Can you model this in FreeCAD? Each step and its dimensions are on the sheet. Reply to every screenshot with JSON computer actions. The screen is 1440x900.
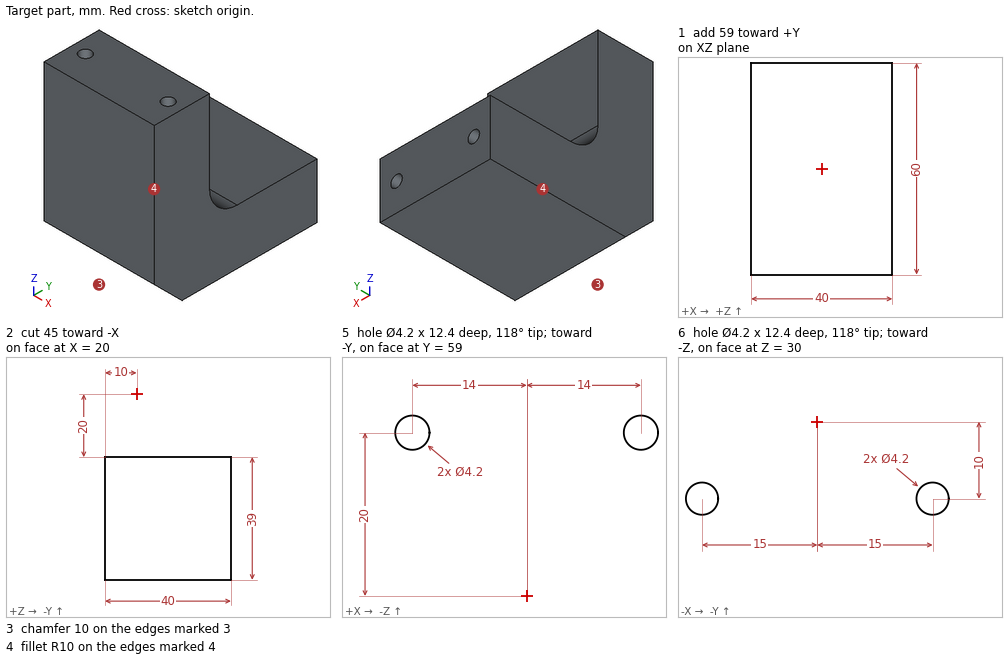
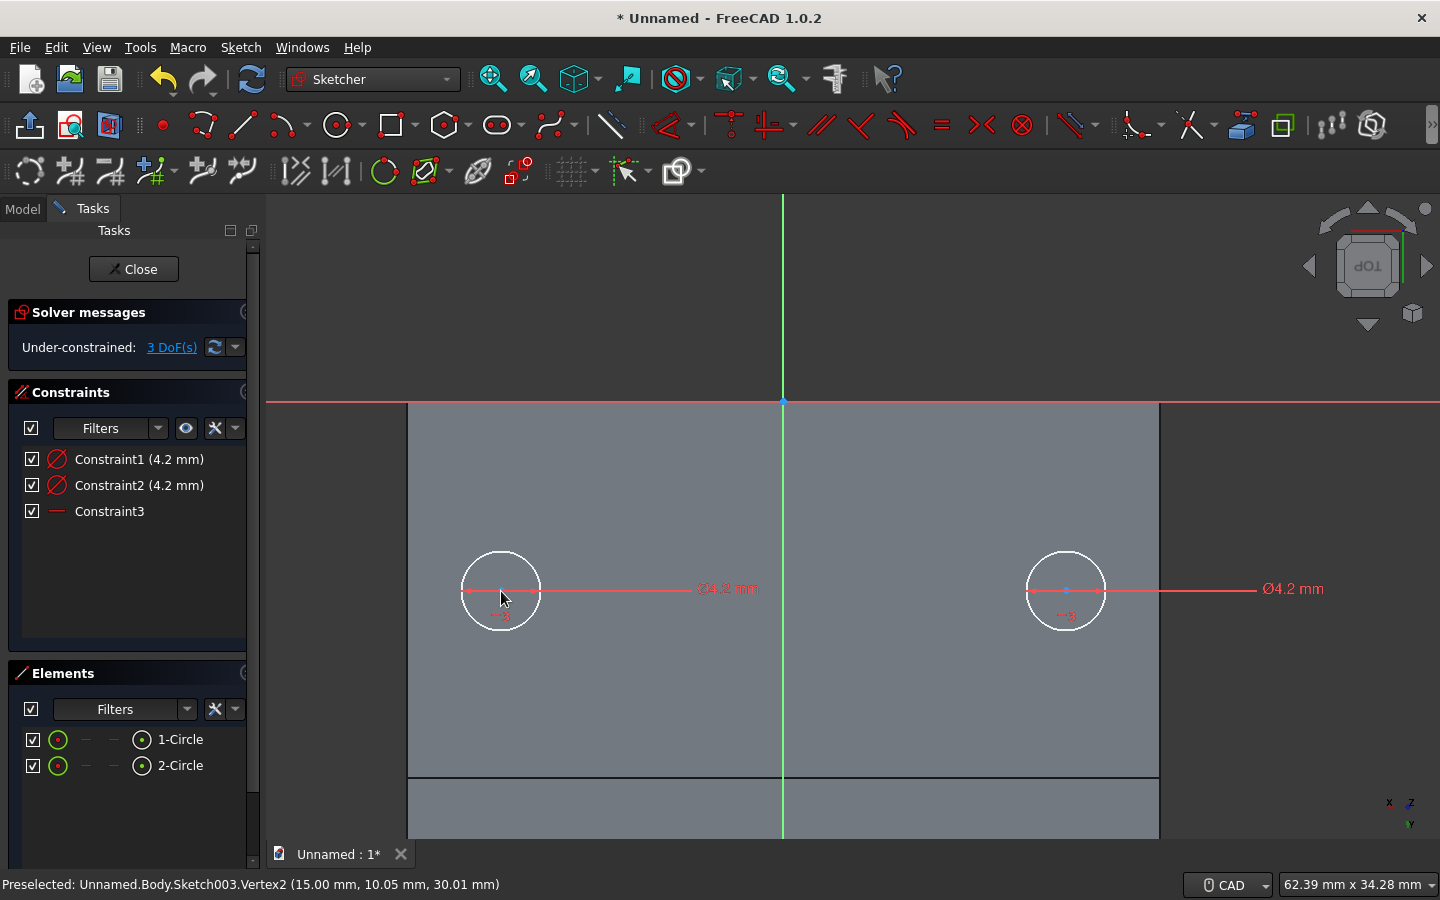
{"action": "left_click", "coordinate": [666, 126]}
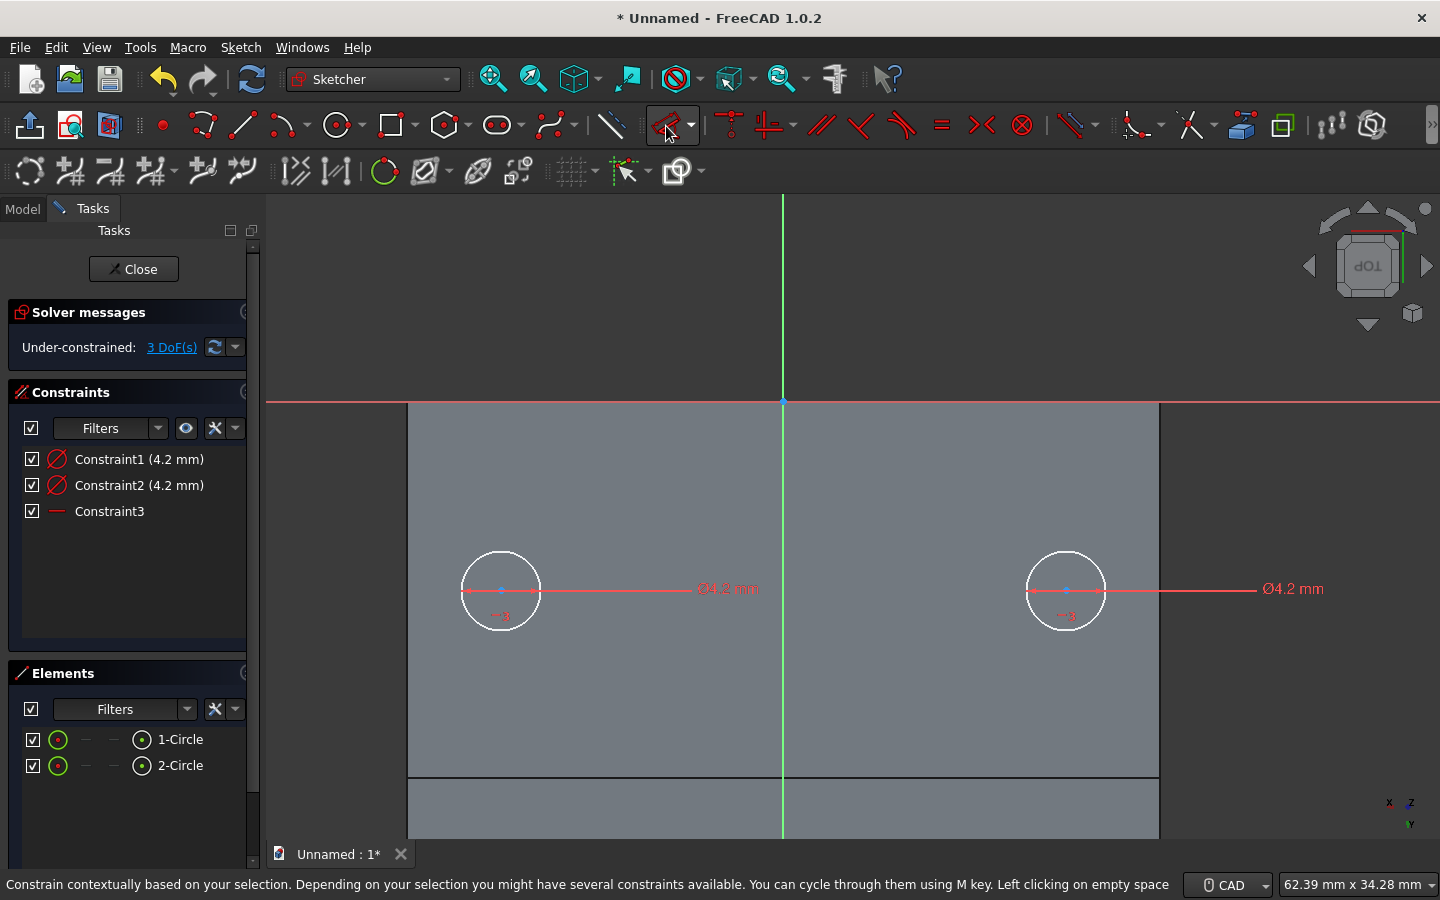
{"action": "left_click", "coordinate": [1066, 591]}
{"action": "left_click", "coordinate": [925, 368]}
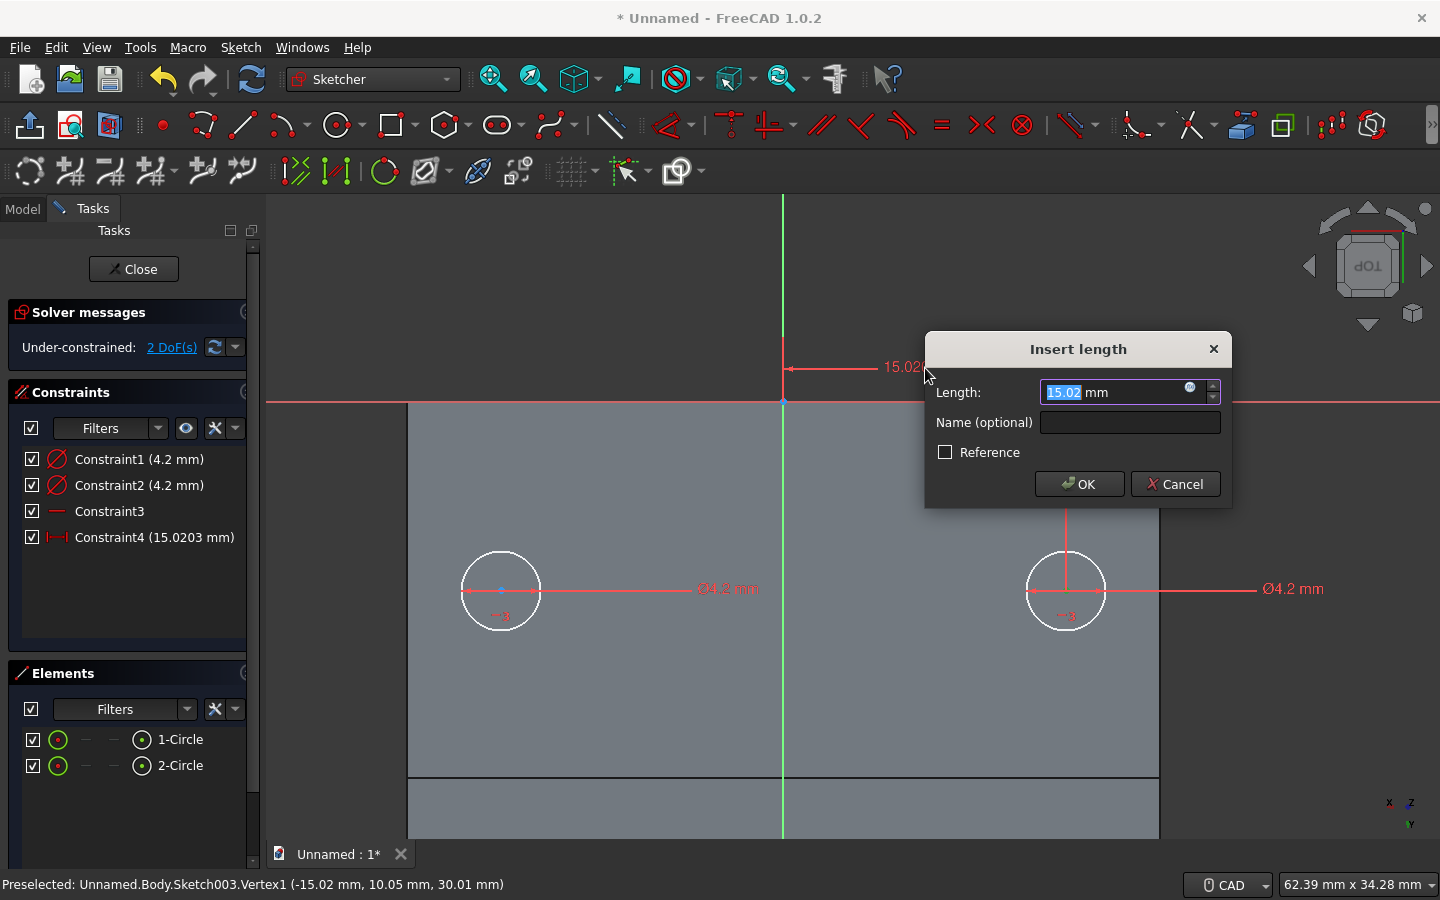
{"action": "type", "text": "15"}
{"action": "key", "text": "Return"}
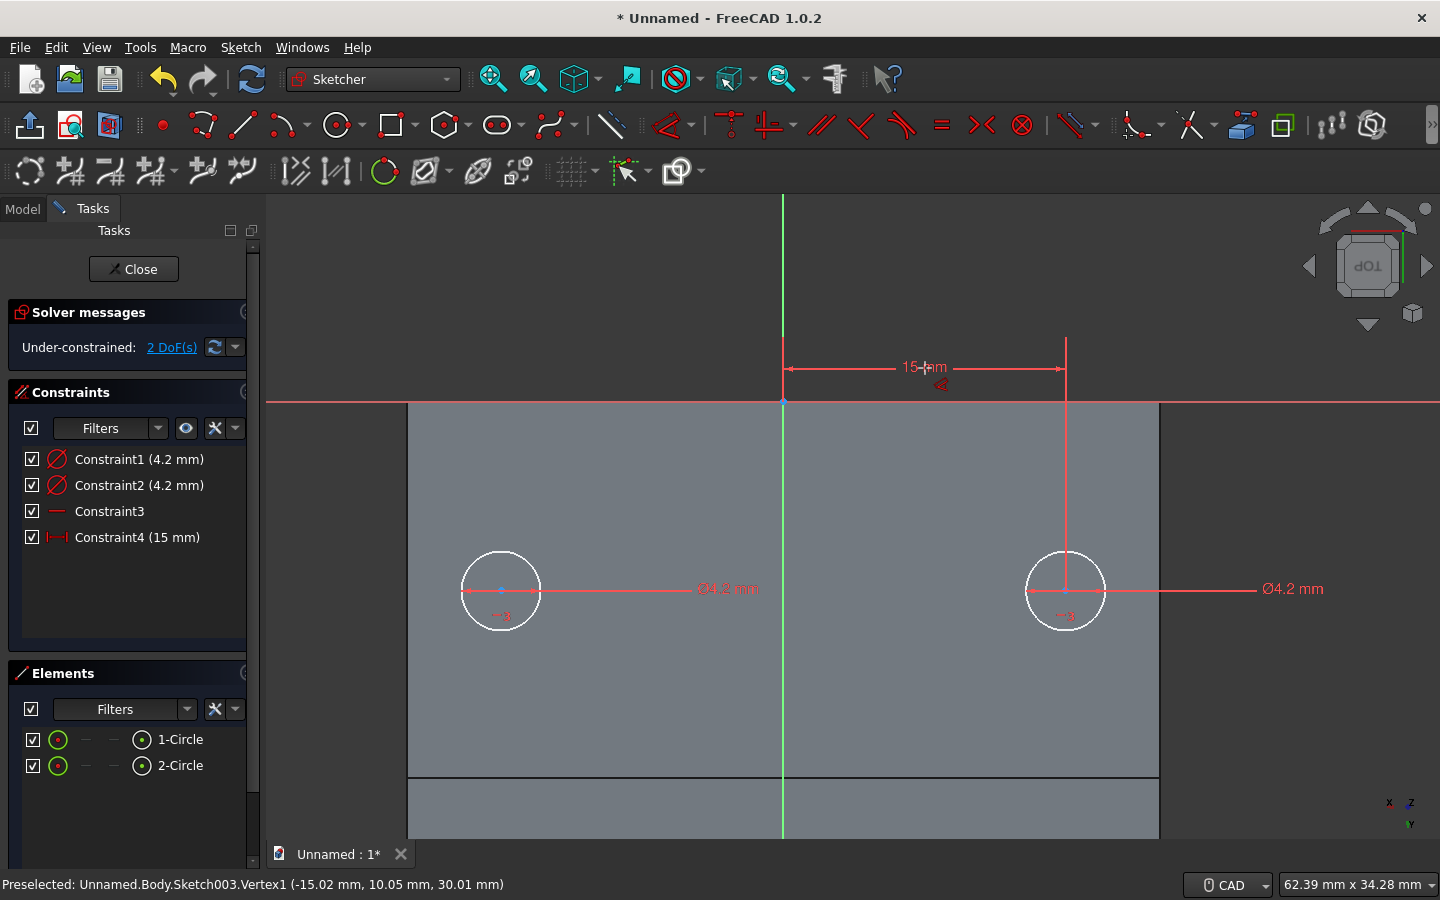
{"action": "left_click", "coordinate": [1066, 591]}
{"action": "left_click", "coordinate": [1100, 496]}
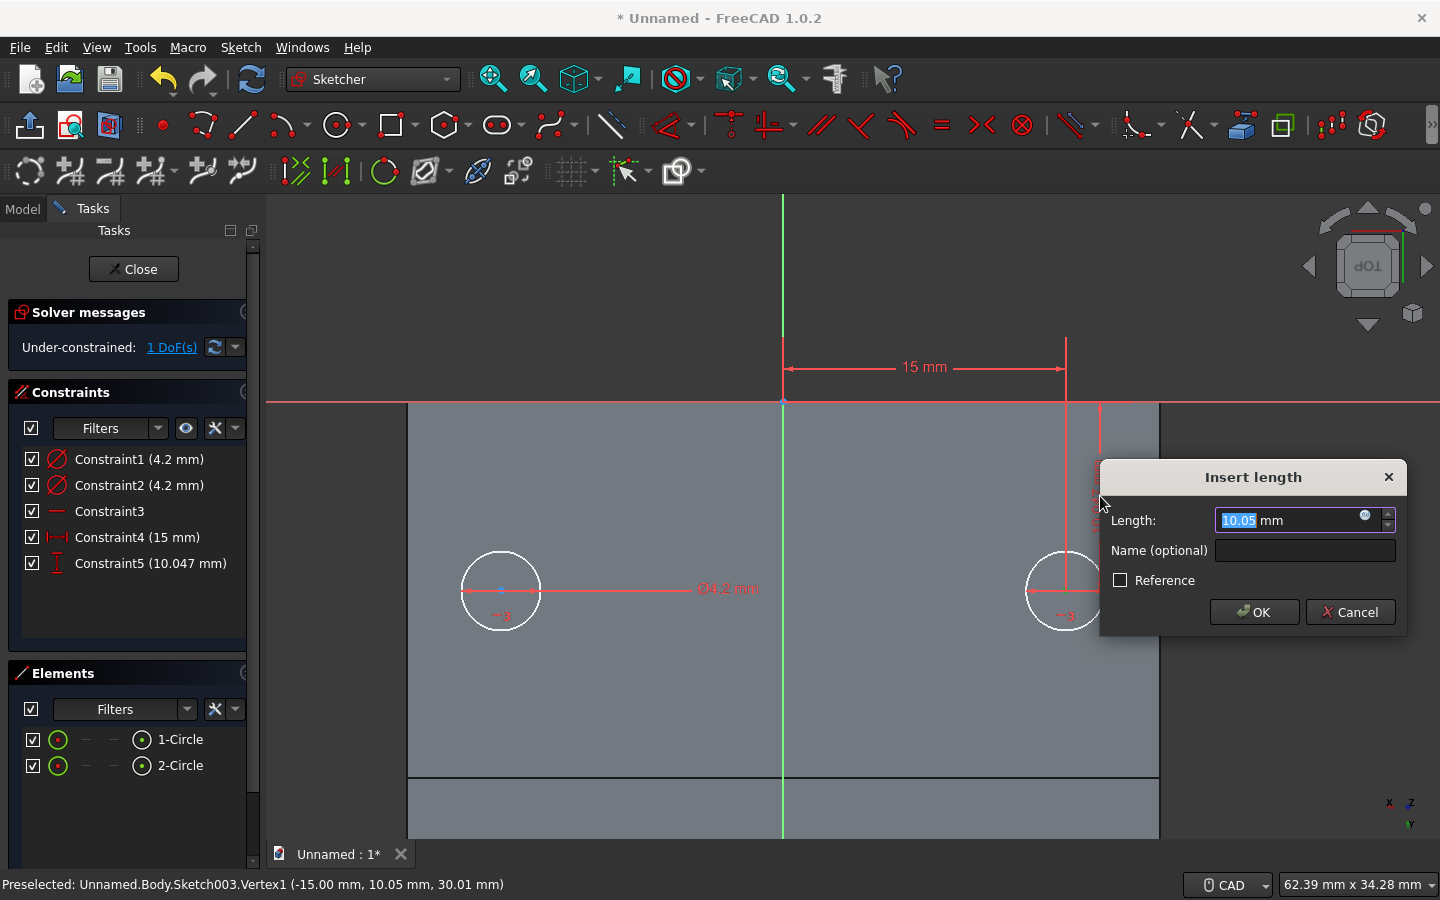
{"action": "type", "text": "10"}
{"action": "key", "text": "Return"}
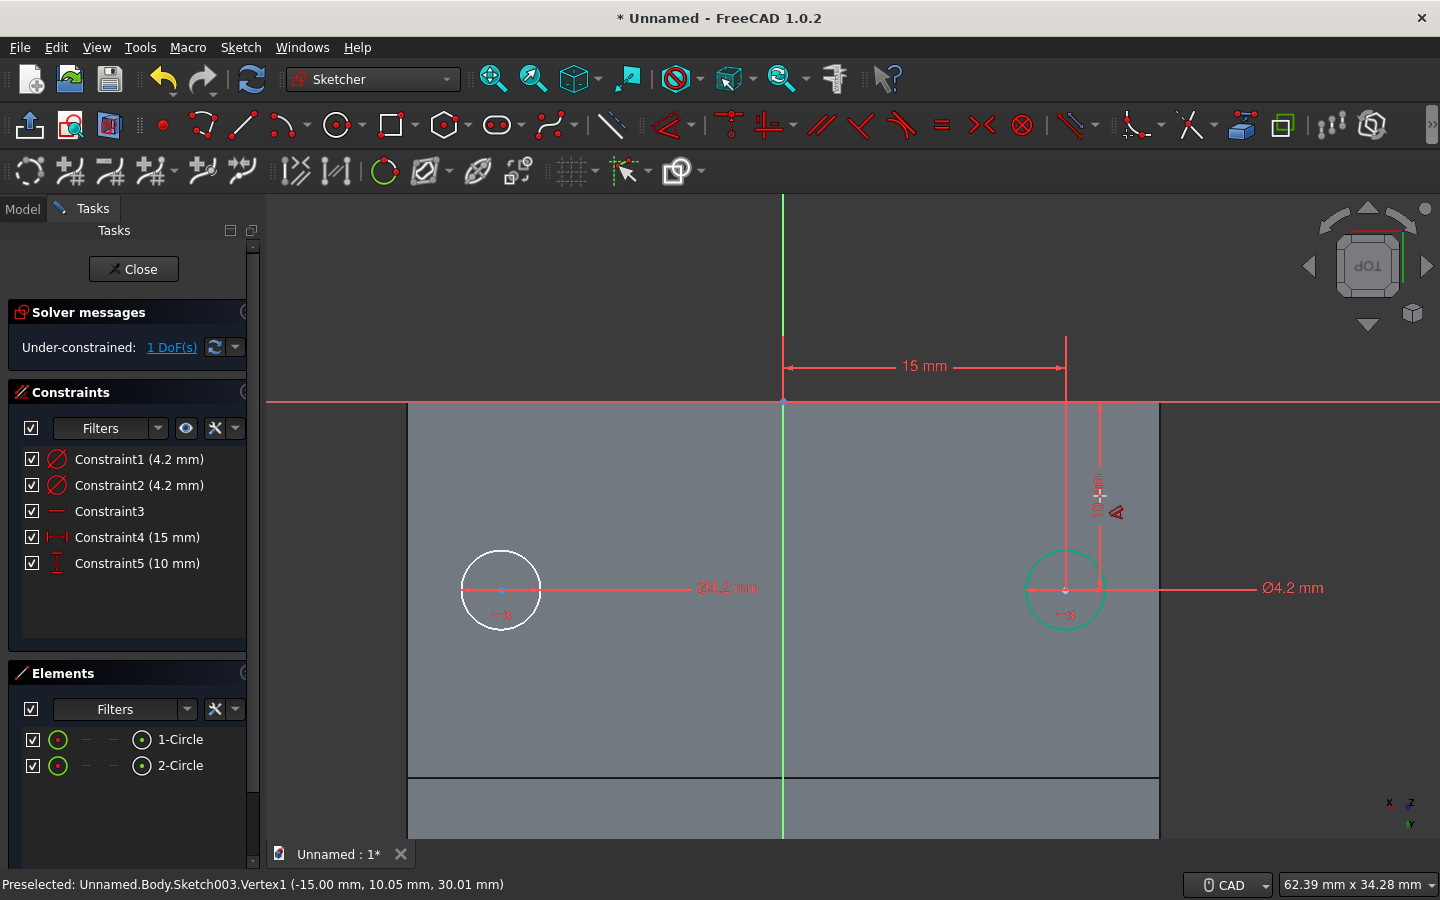
{"action": "left_click", "coordinate": [501, 590]}
{"action": "left_click", "coordinate": [642, 368]}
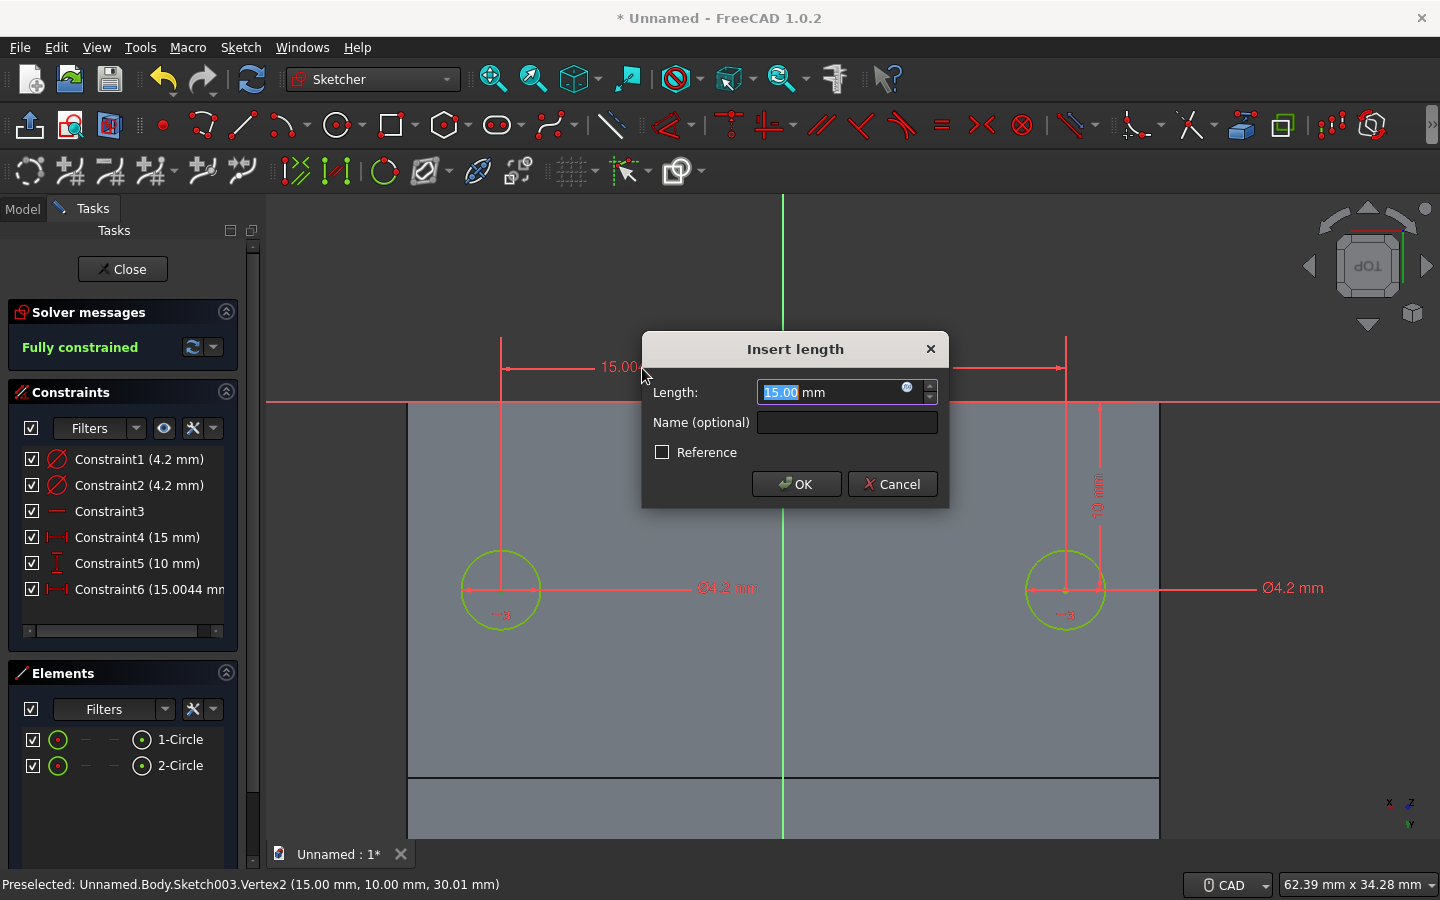
{"action": "type", "text": "15"}
{"action": "key", "text": "Return"}
{"action": "key", "text": "Escape"}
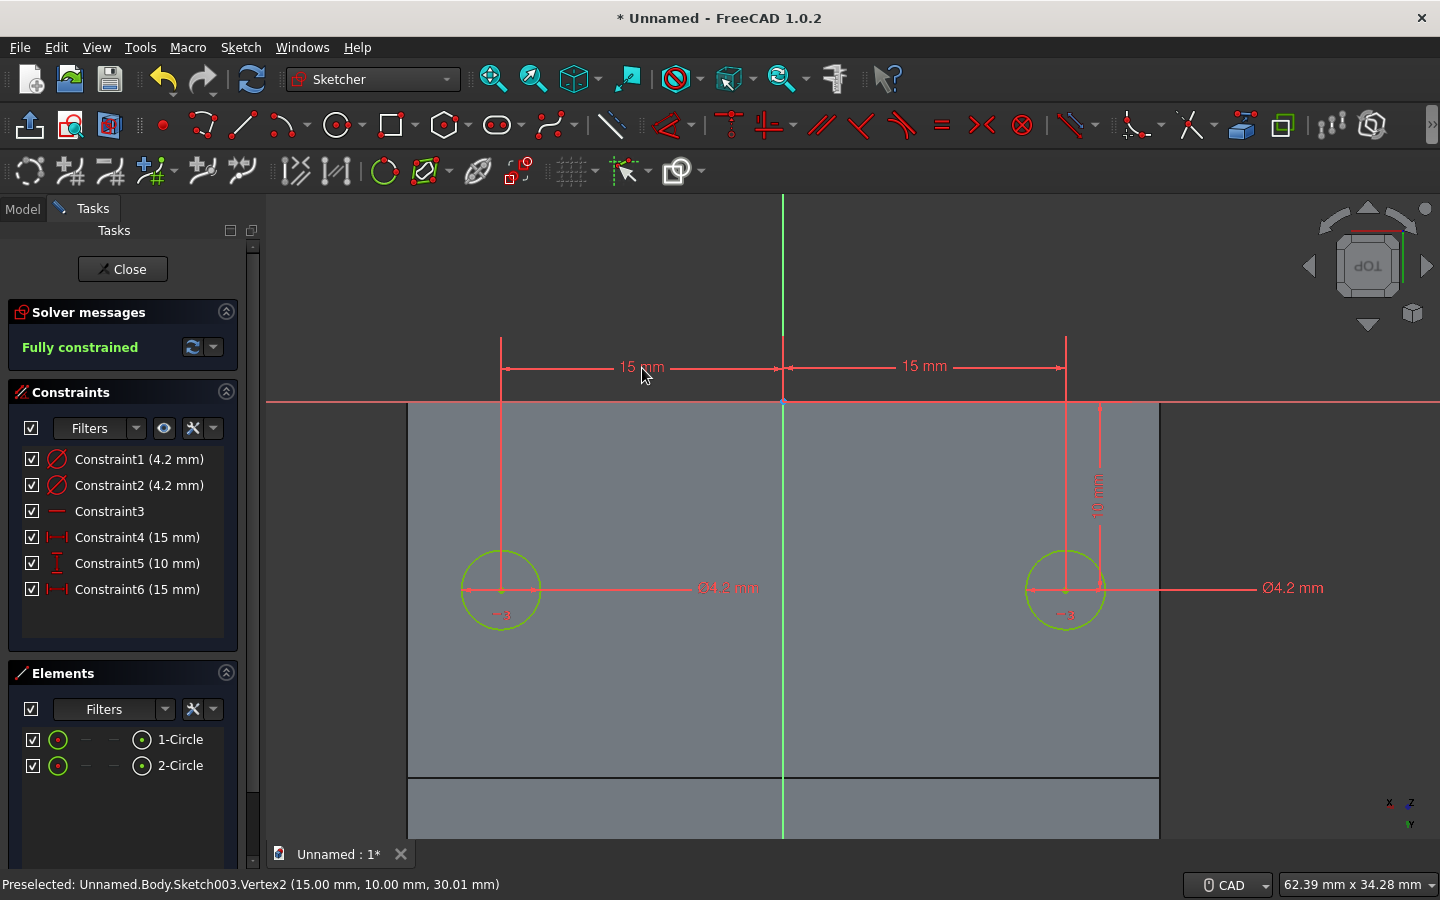
{"action": "left_click", "coordinate": [123, 269]}